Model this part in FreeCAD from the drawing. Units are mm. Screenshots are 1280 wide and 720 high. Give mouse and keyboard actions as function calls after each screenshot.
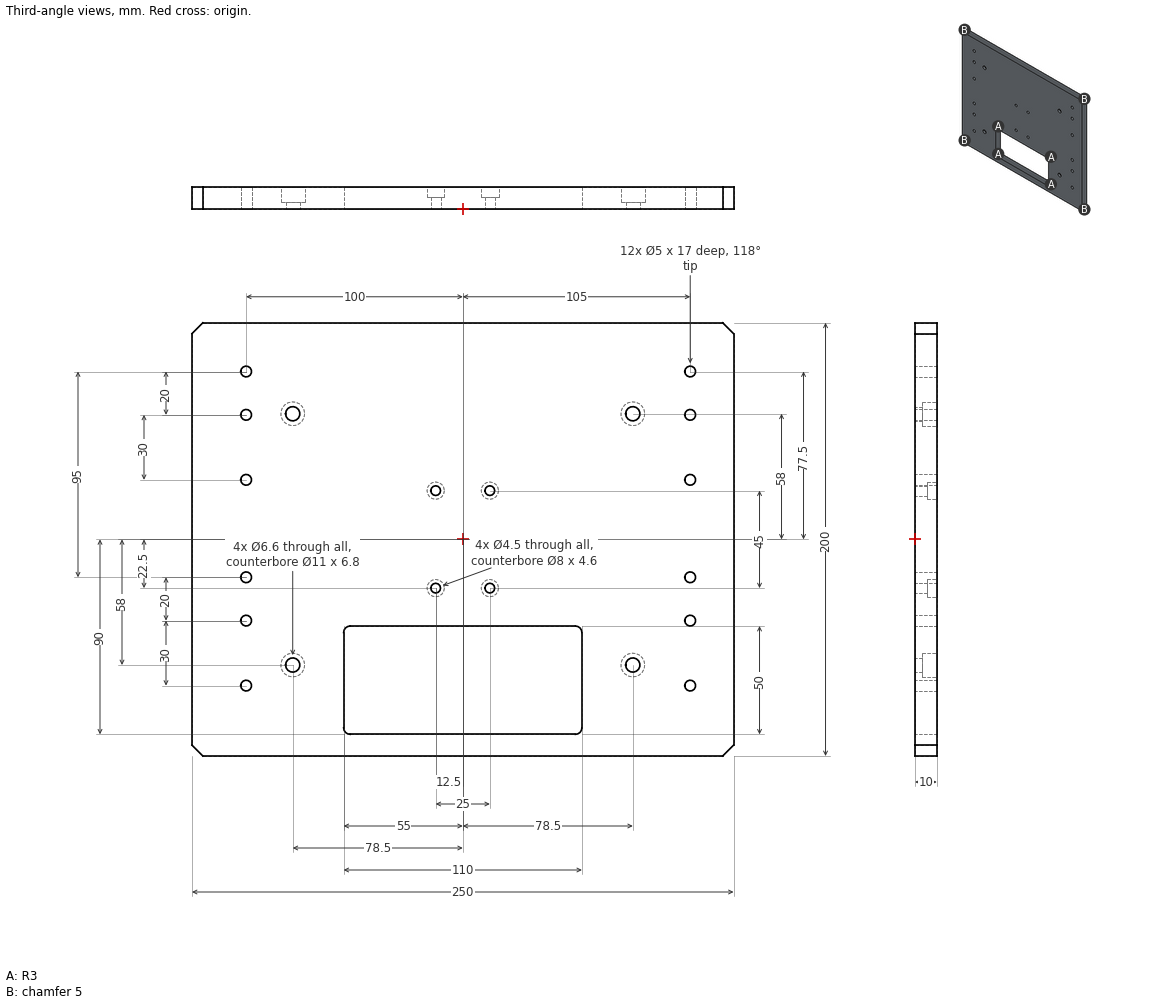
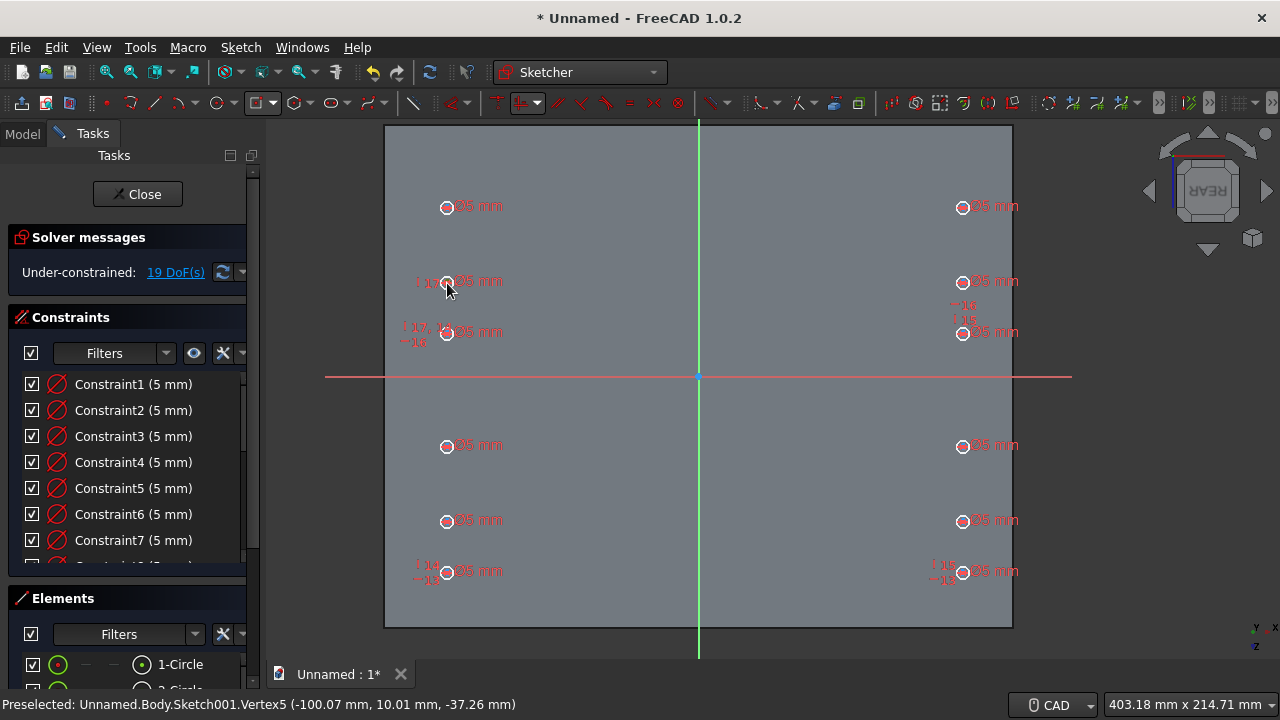
click(447, 208)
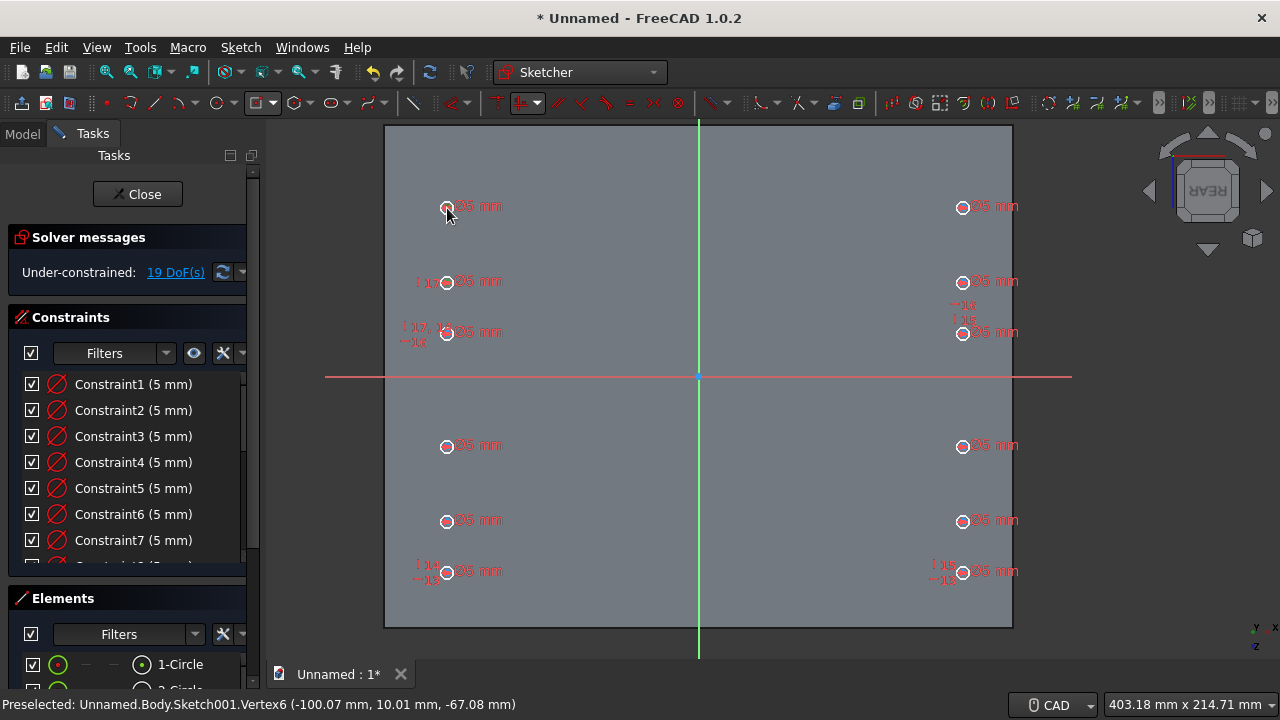
key(v)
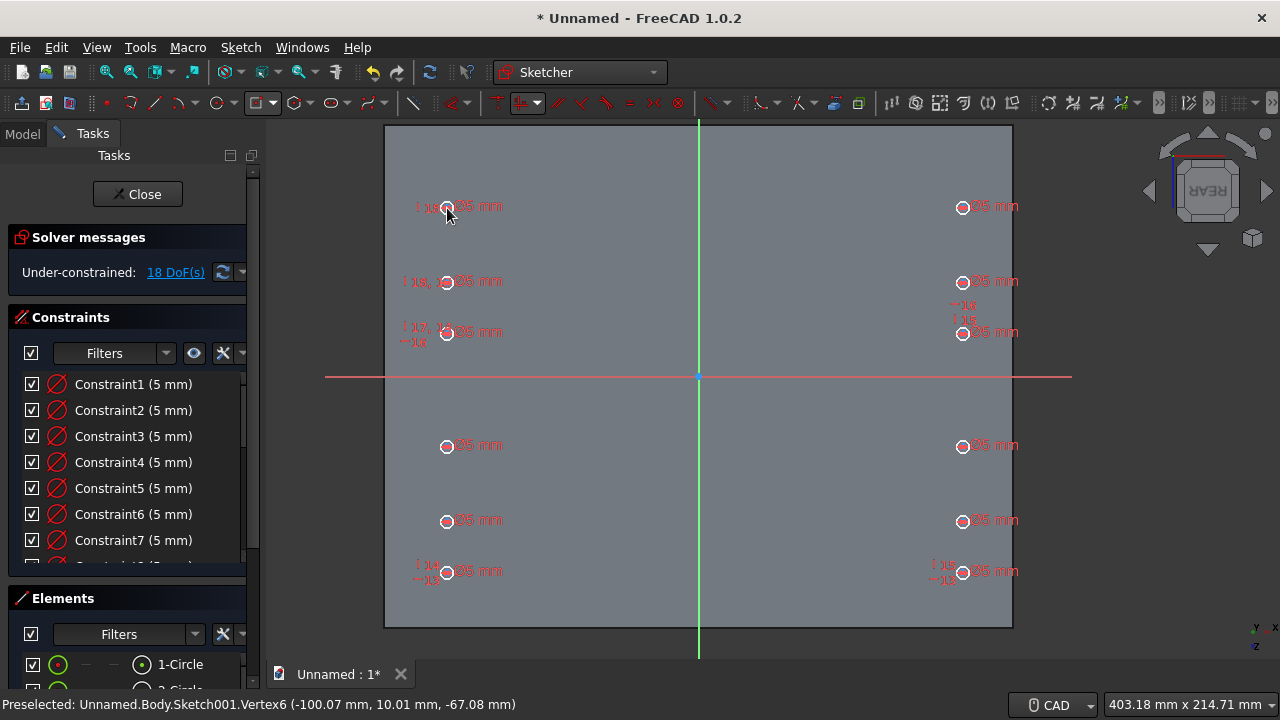
click(963, 334)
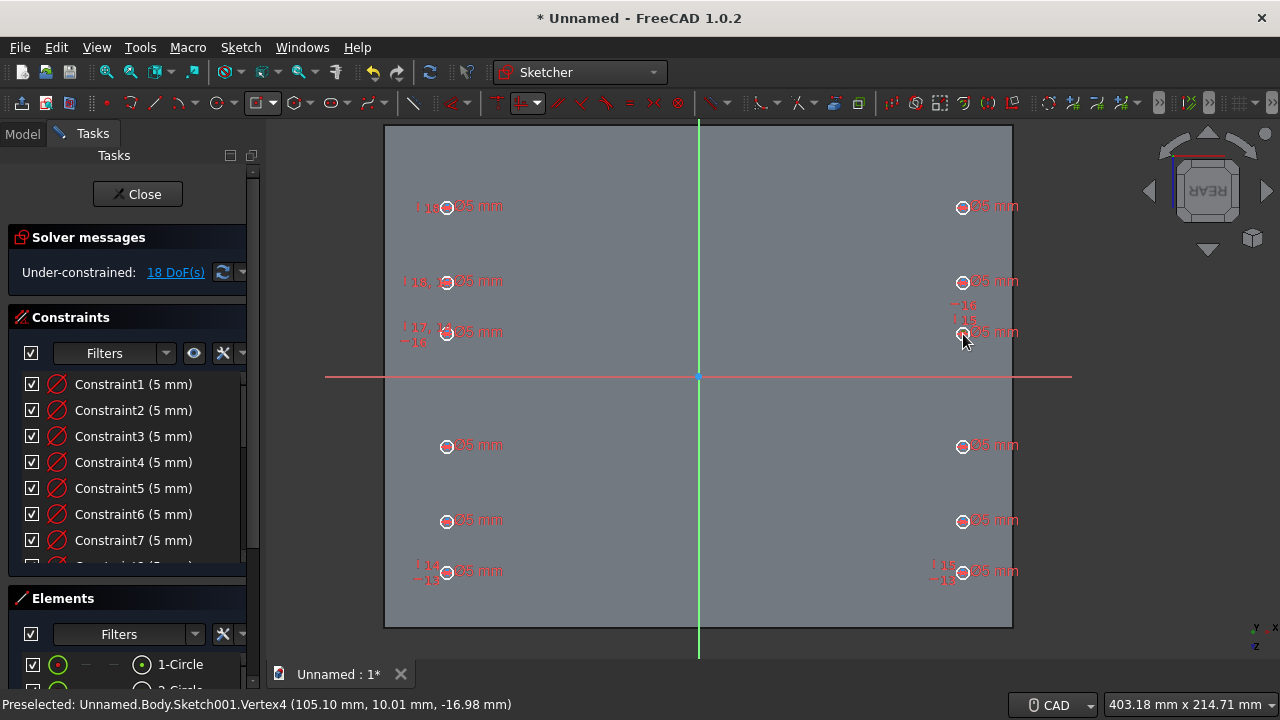
click(963, 283)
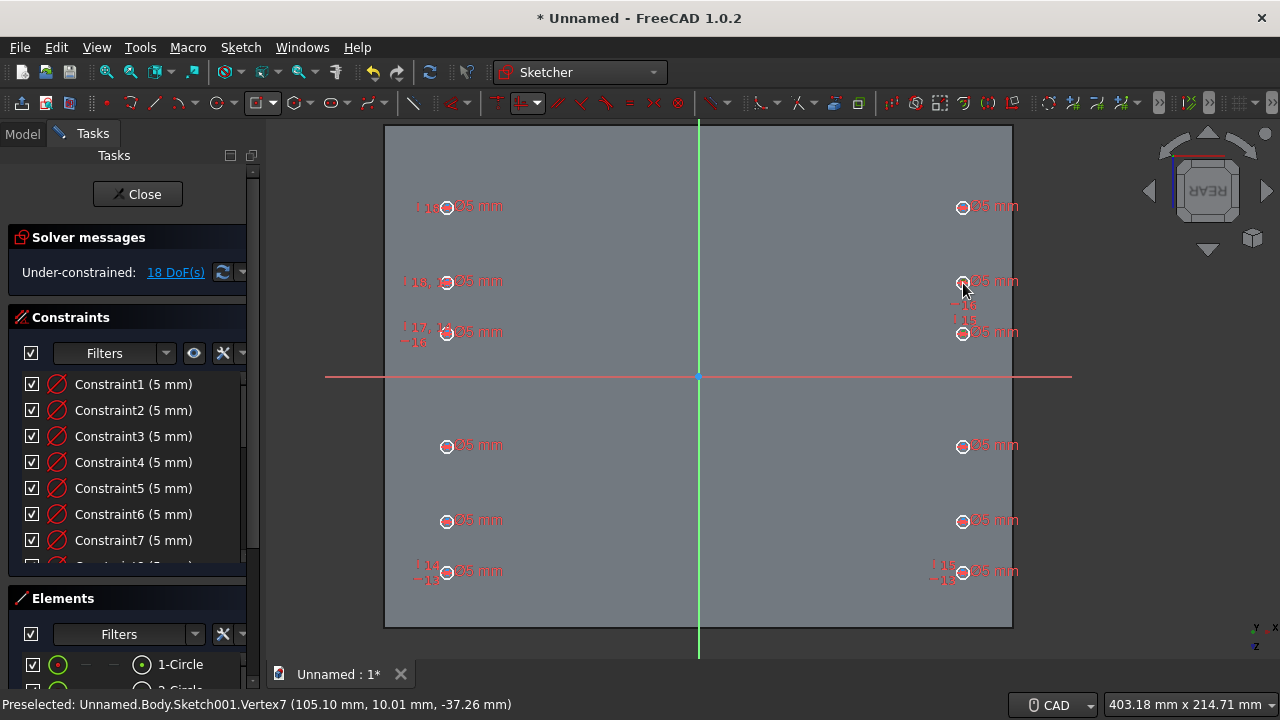
click(540, 104)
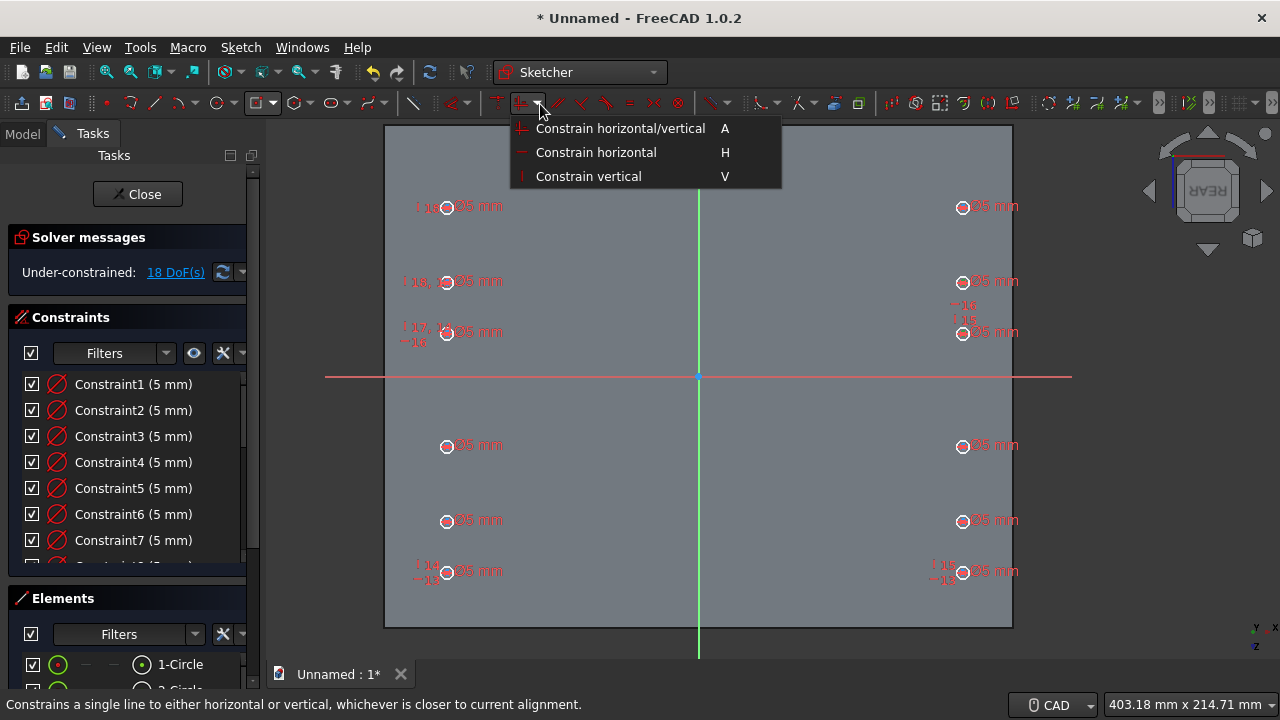
click(646, 176)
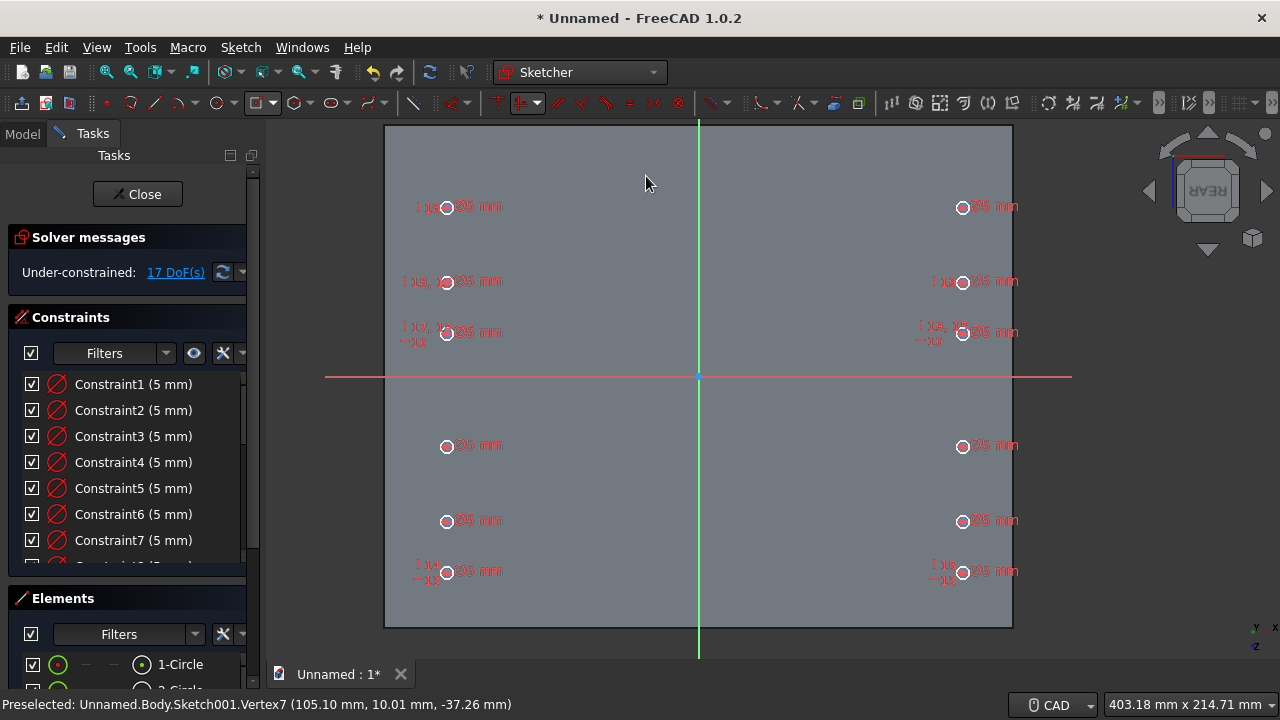
click(447, 283)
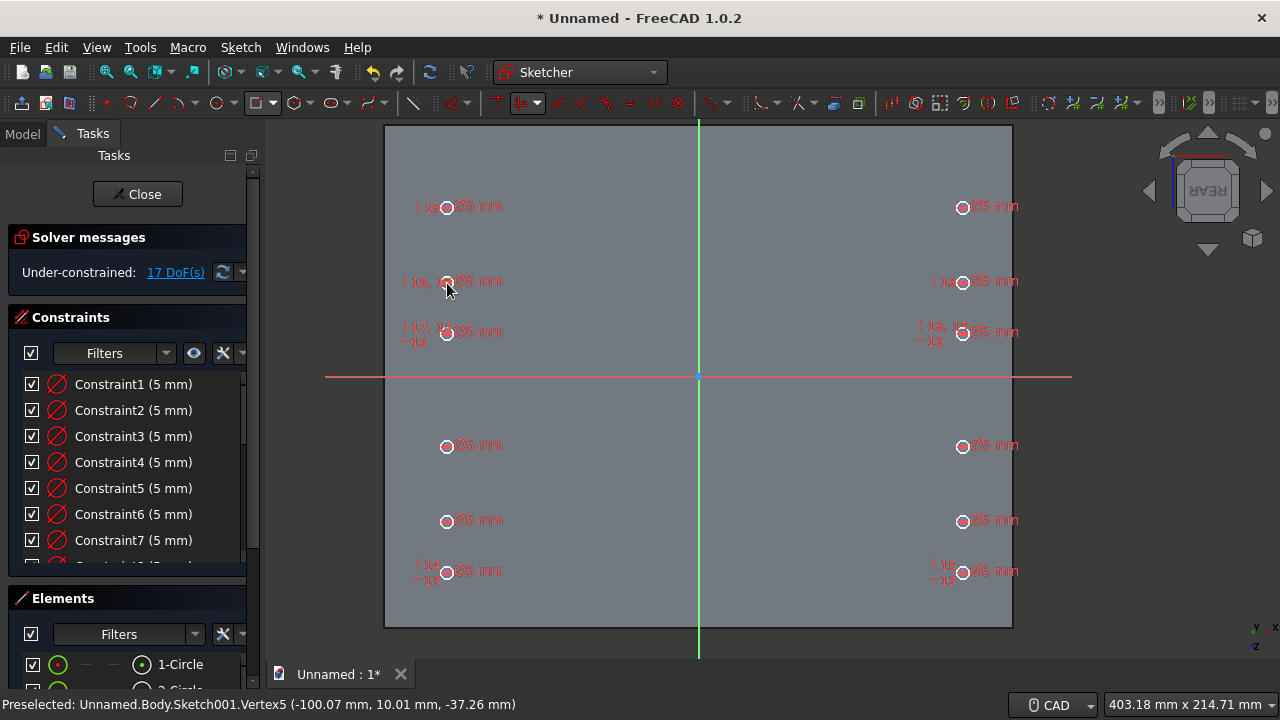
click(963, 283)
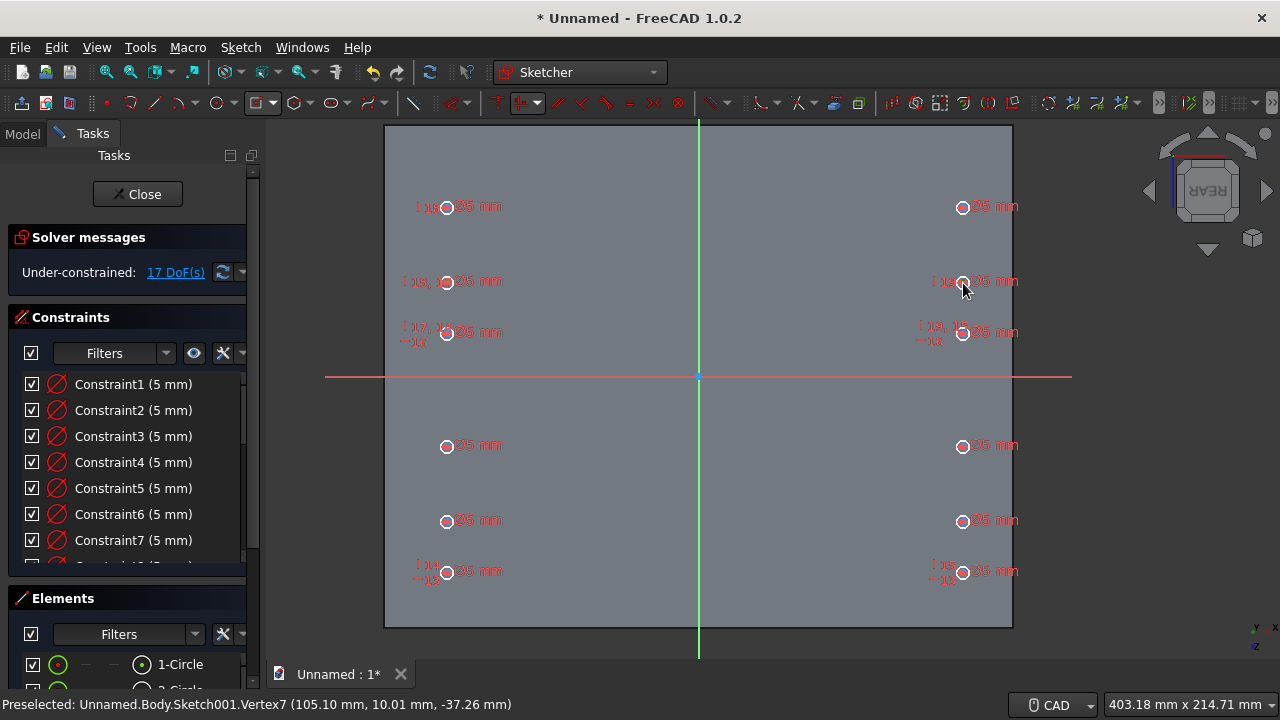
key(h)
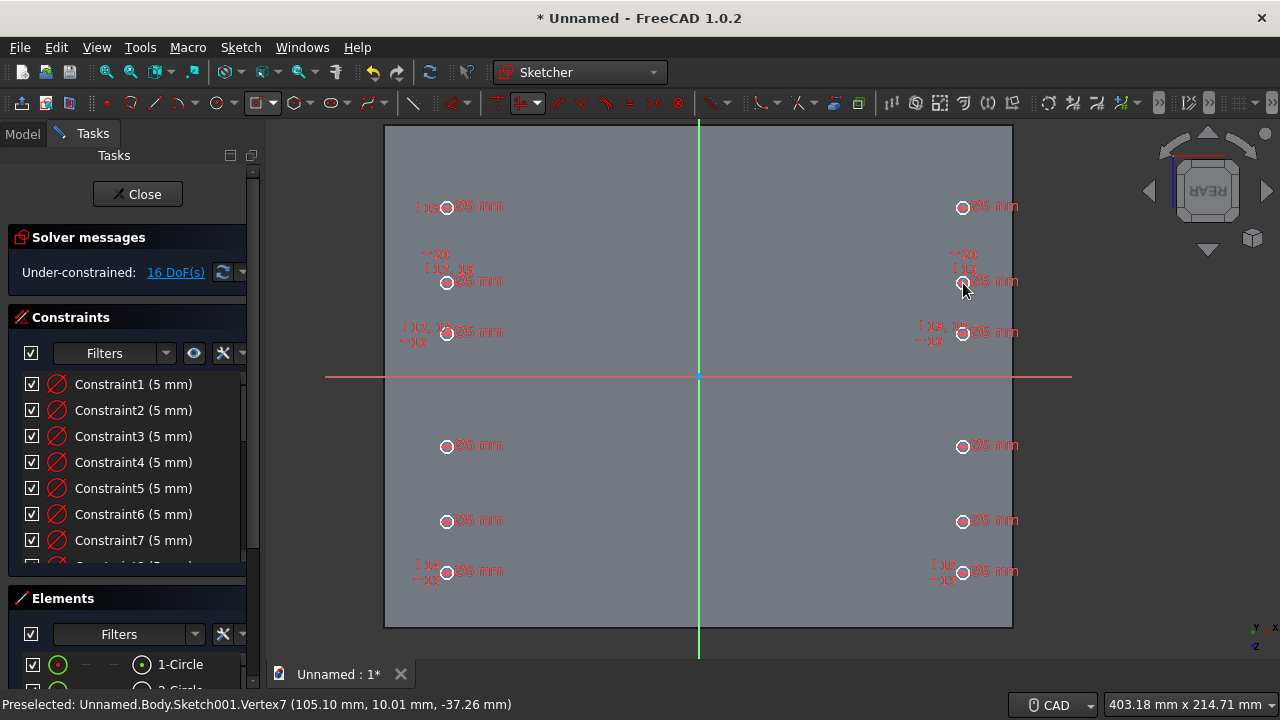
click(963, 283)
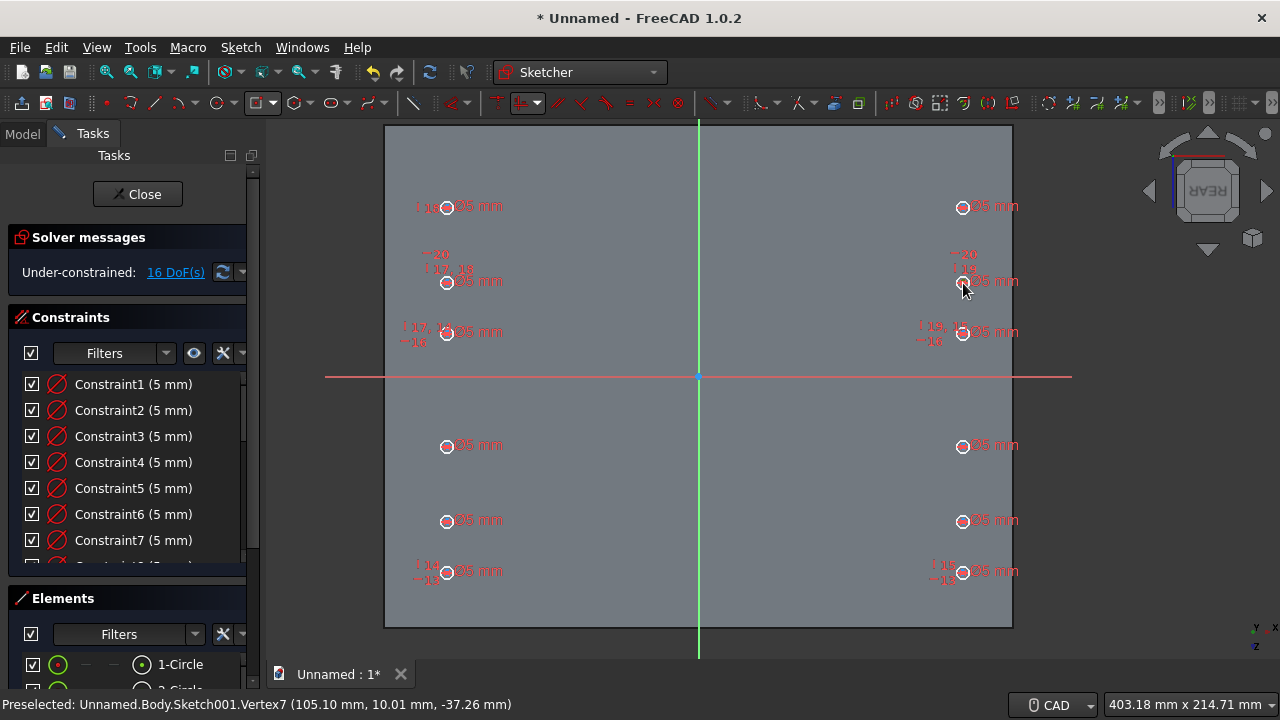
click(963, 208)